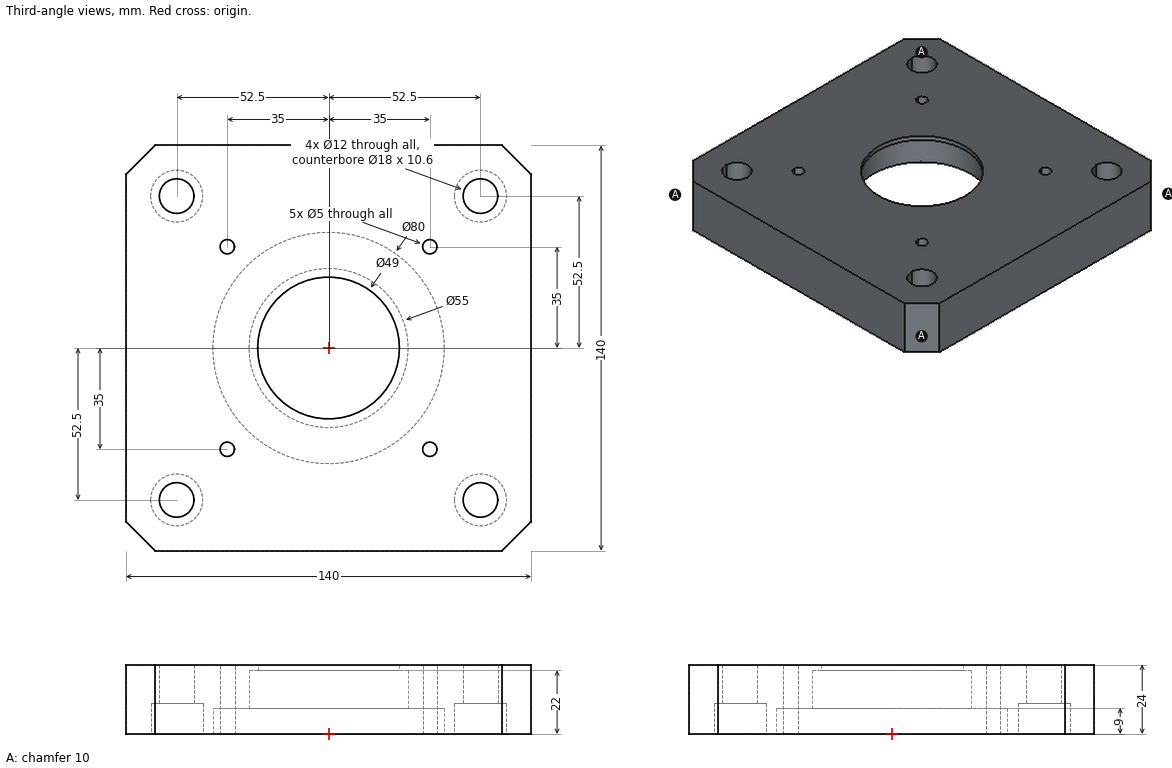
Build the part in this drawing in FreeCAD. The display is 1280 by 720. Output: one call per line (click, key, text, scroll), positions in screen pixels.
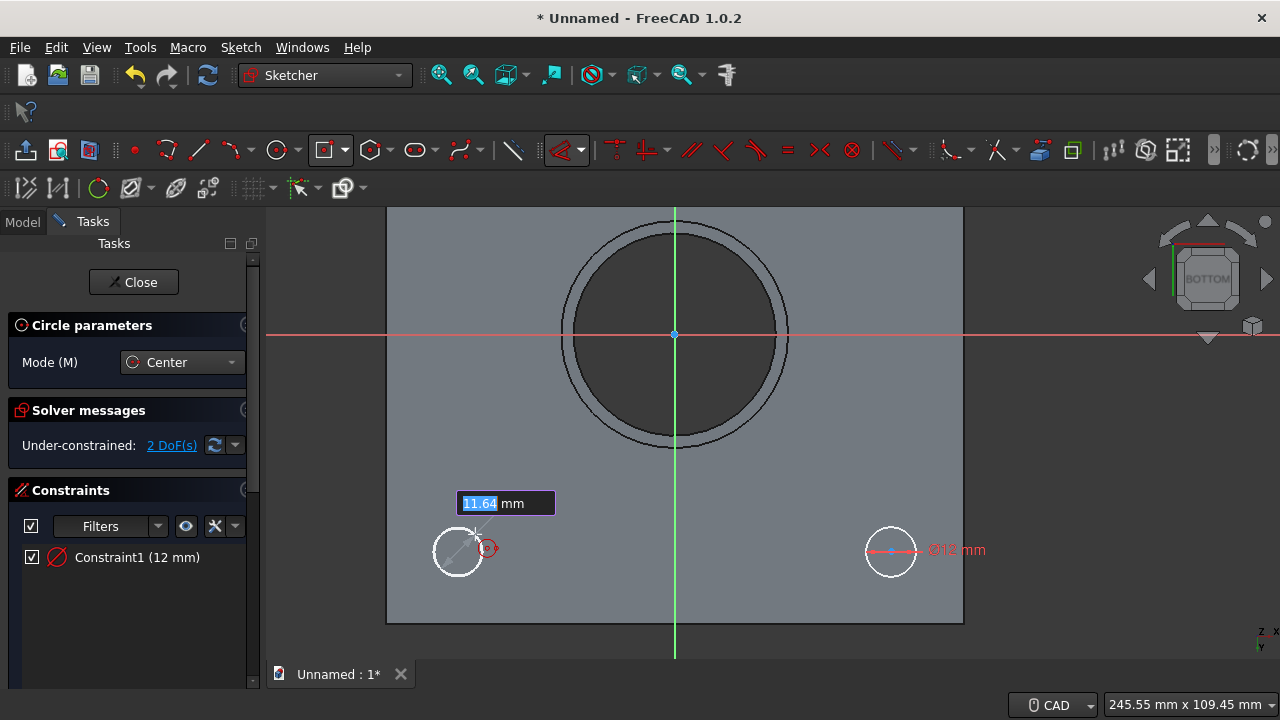
text(12)
key(Return)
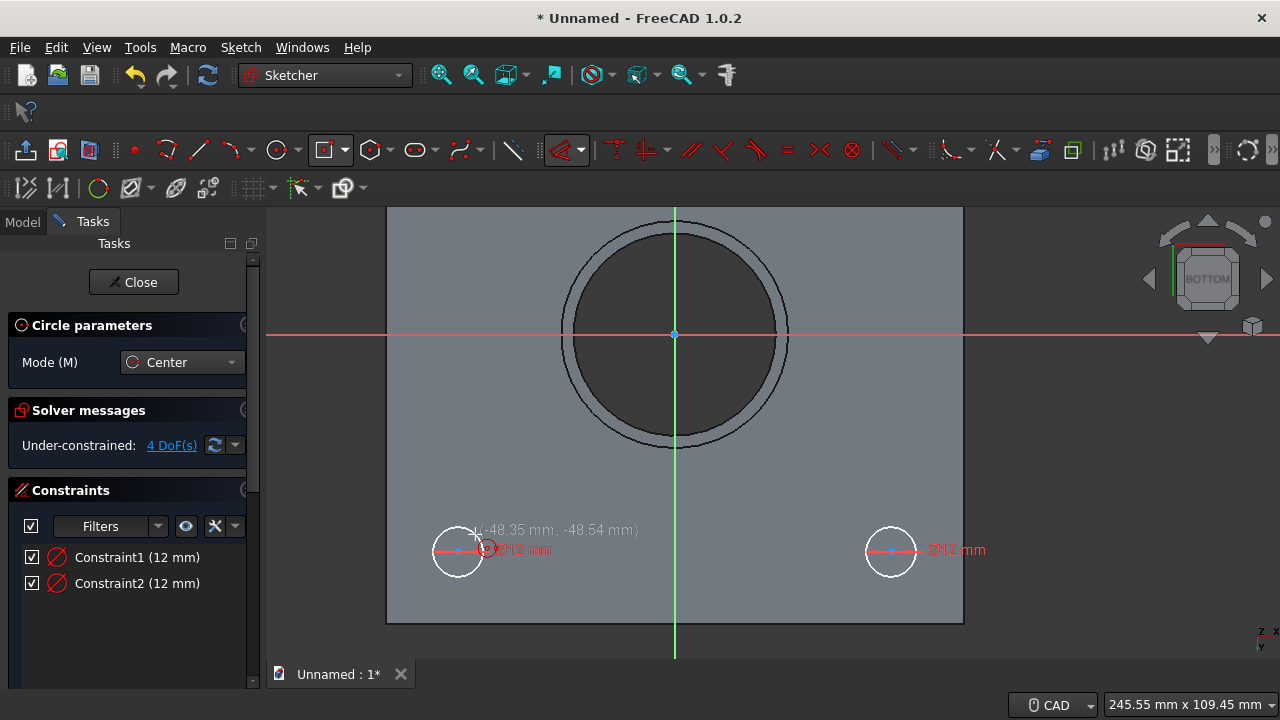
scroll(741, 553, down, 3)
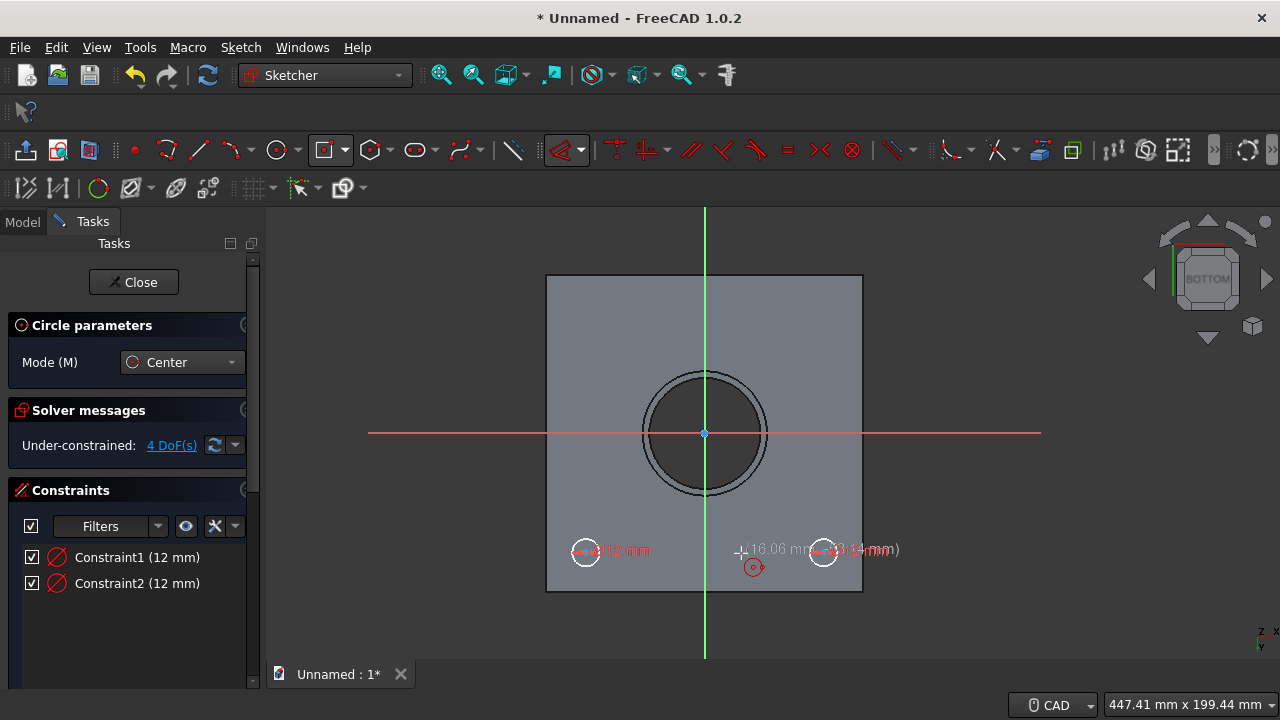
scroll(586, 314, up, 3)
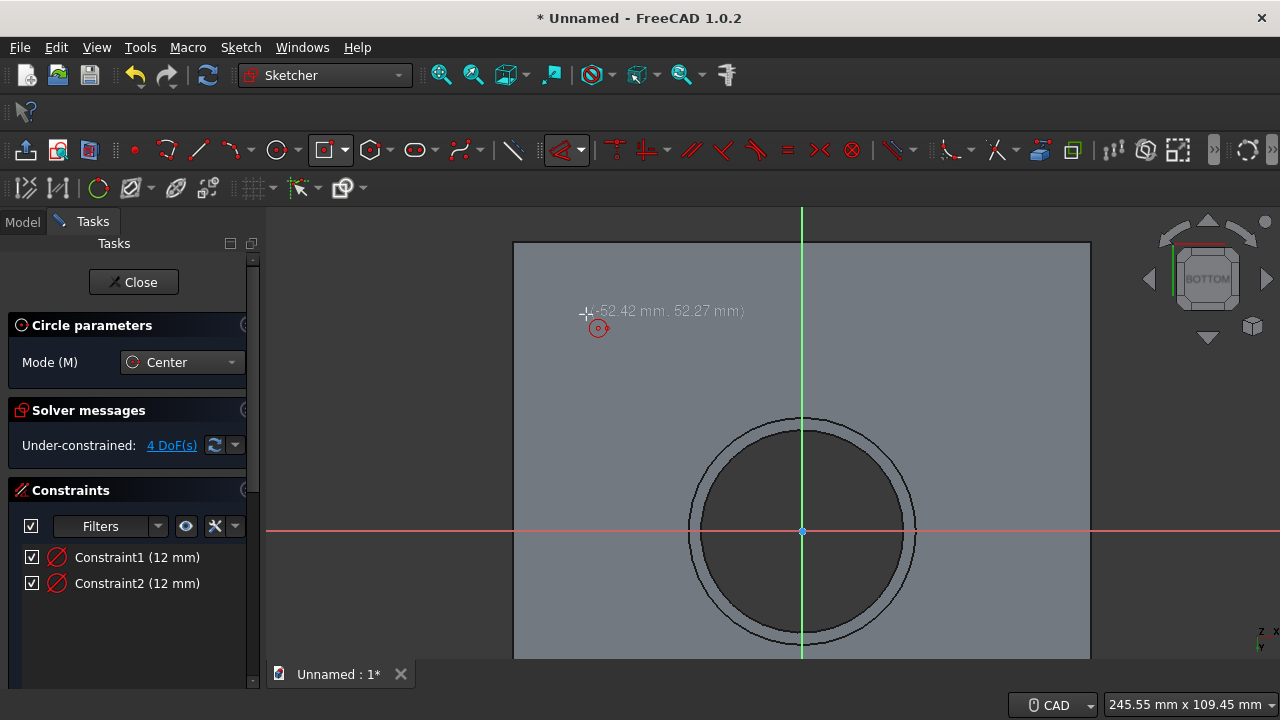
click(585, 315)
move(603, 297)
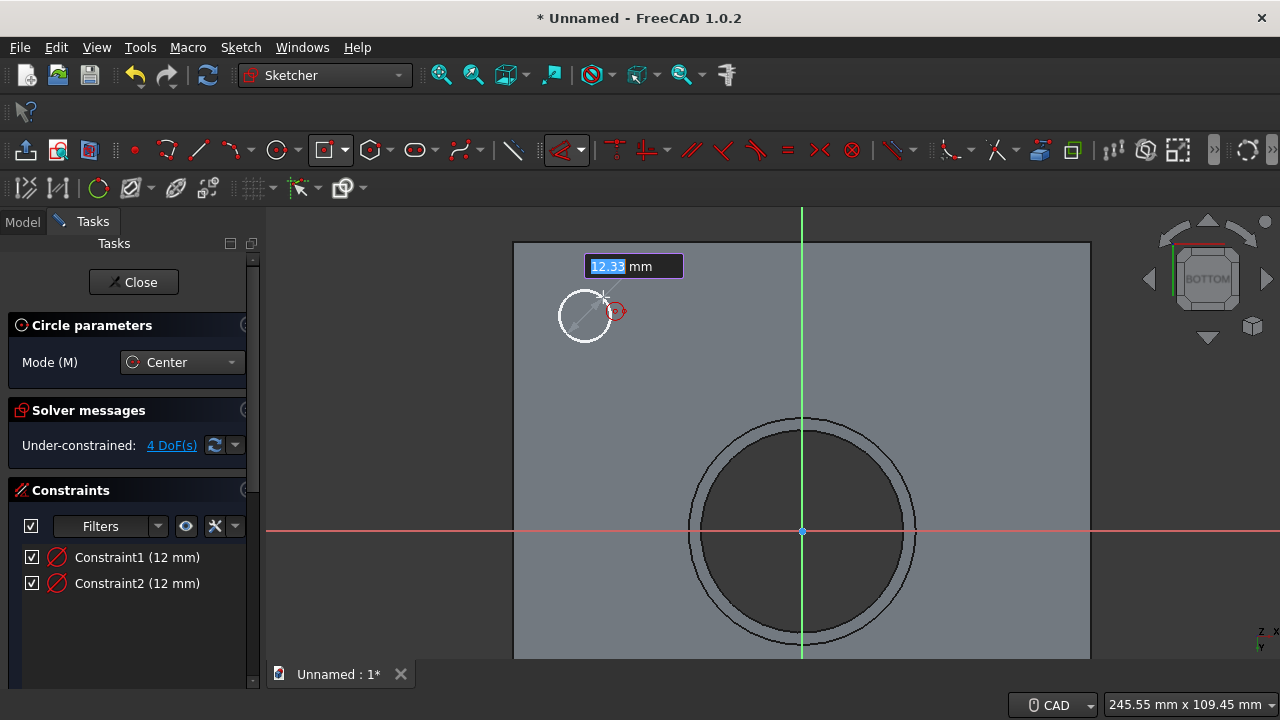
text(12)
key(Return)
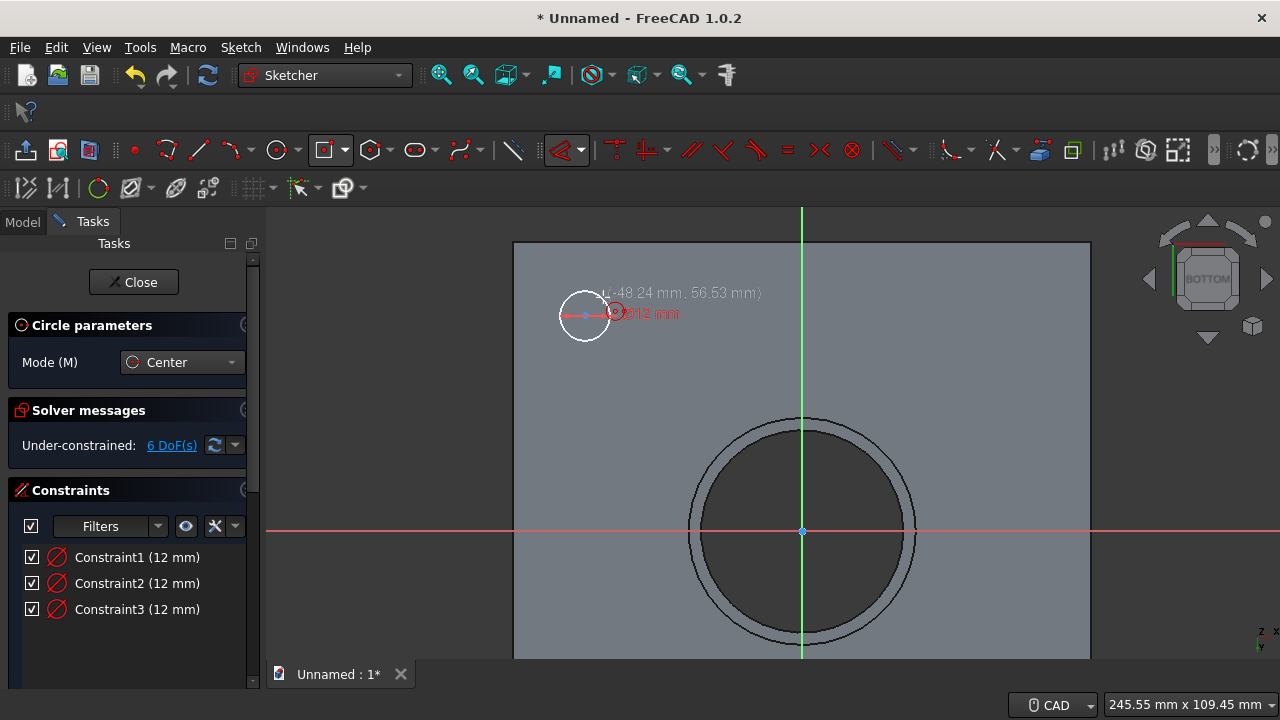
click(1019, 315)
move(1037, 297)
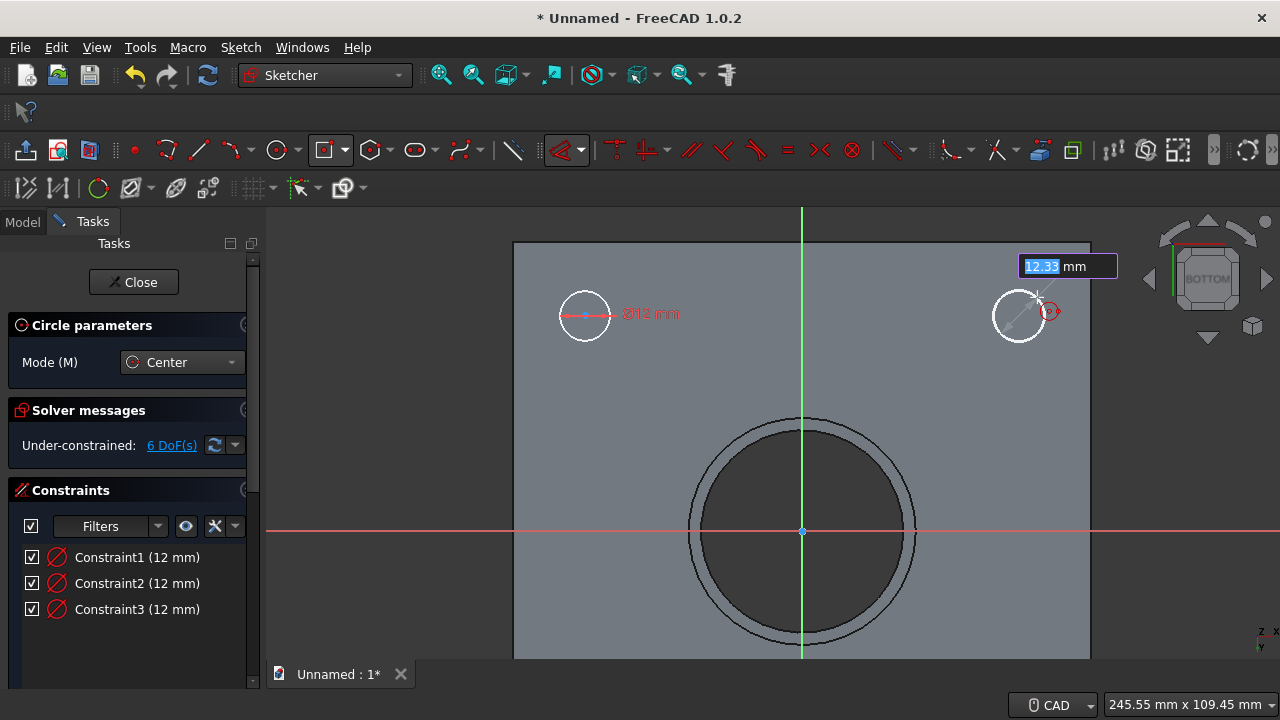
text(12)
key(Return)
key(Escape)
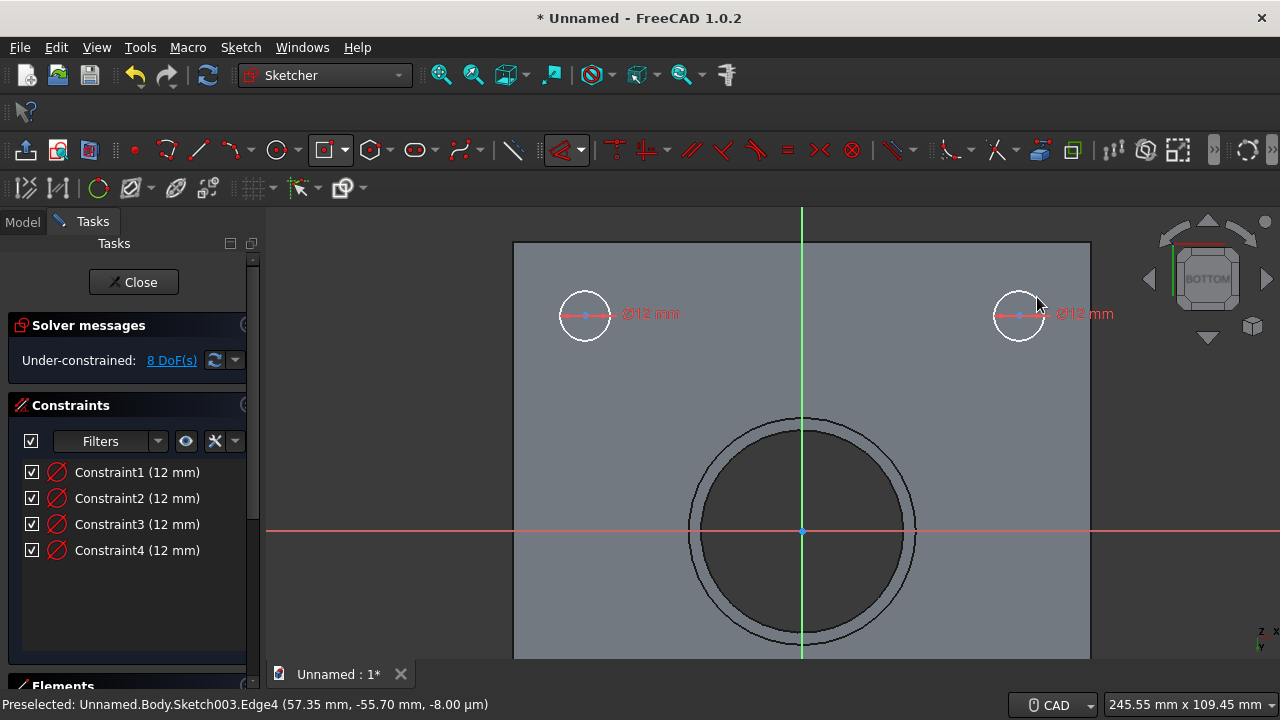
scroll(586, 313, down, 3)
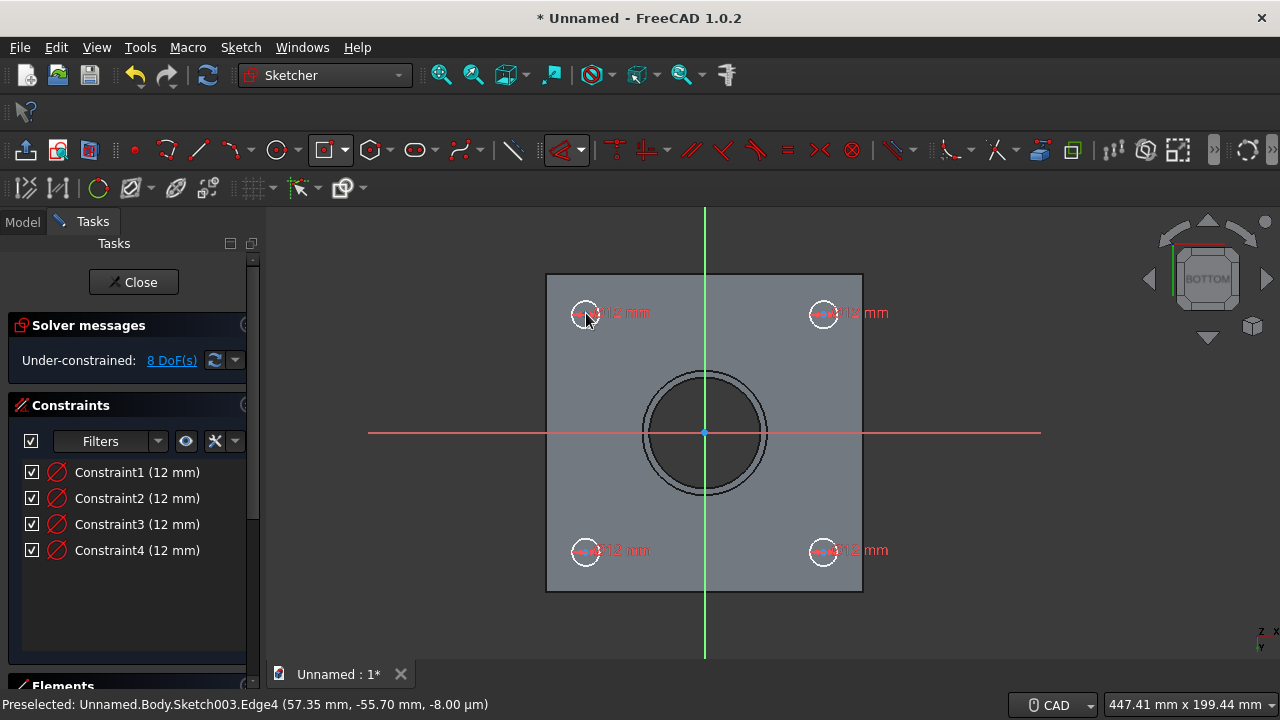
click(824, 552)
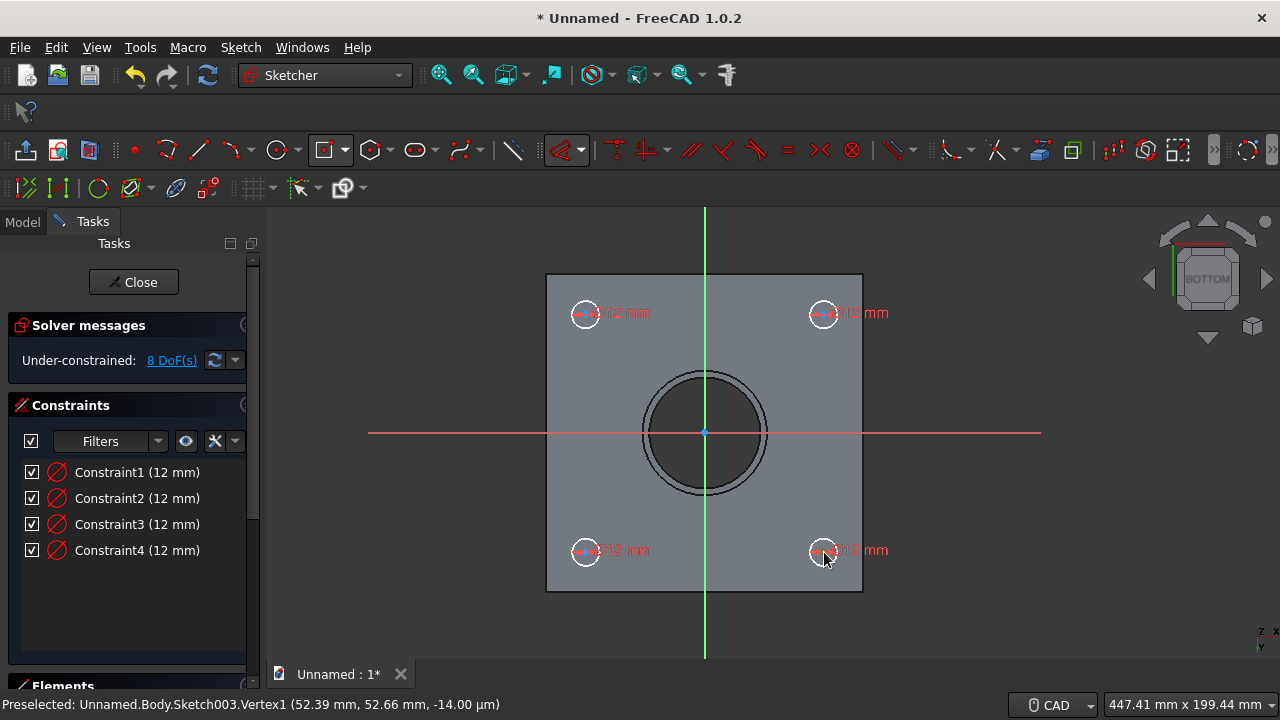
click(586, 552)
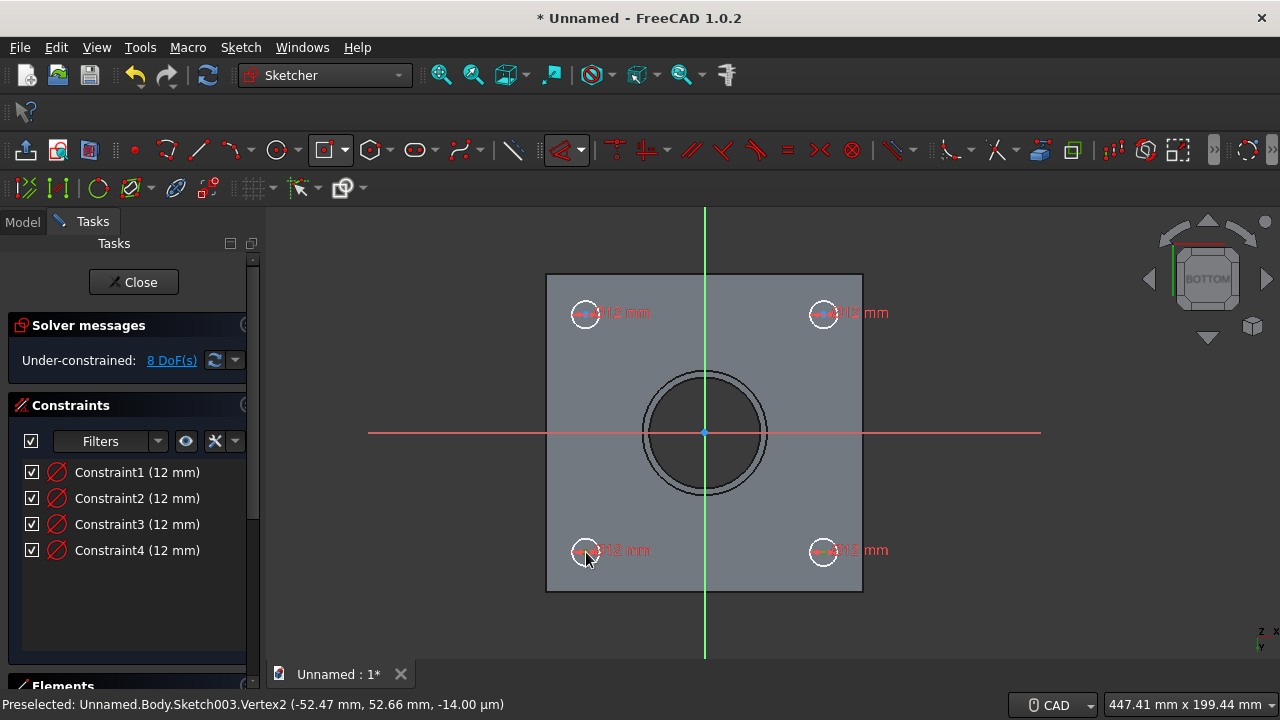
click(670, 150)